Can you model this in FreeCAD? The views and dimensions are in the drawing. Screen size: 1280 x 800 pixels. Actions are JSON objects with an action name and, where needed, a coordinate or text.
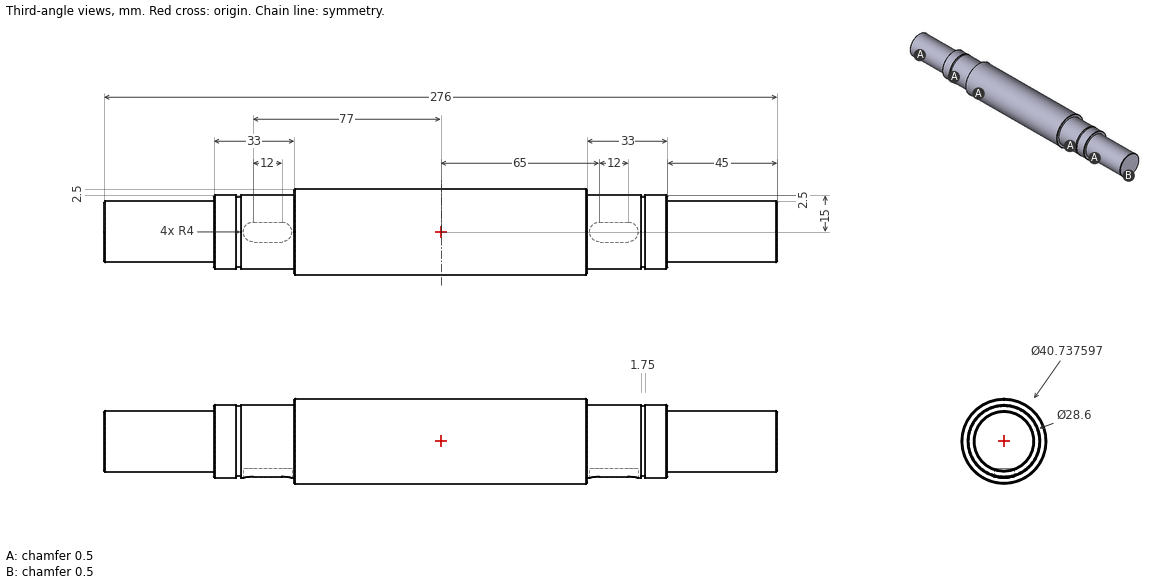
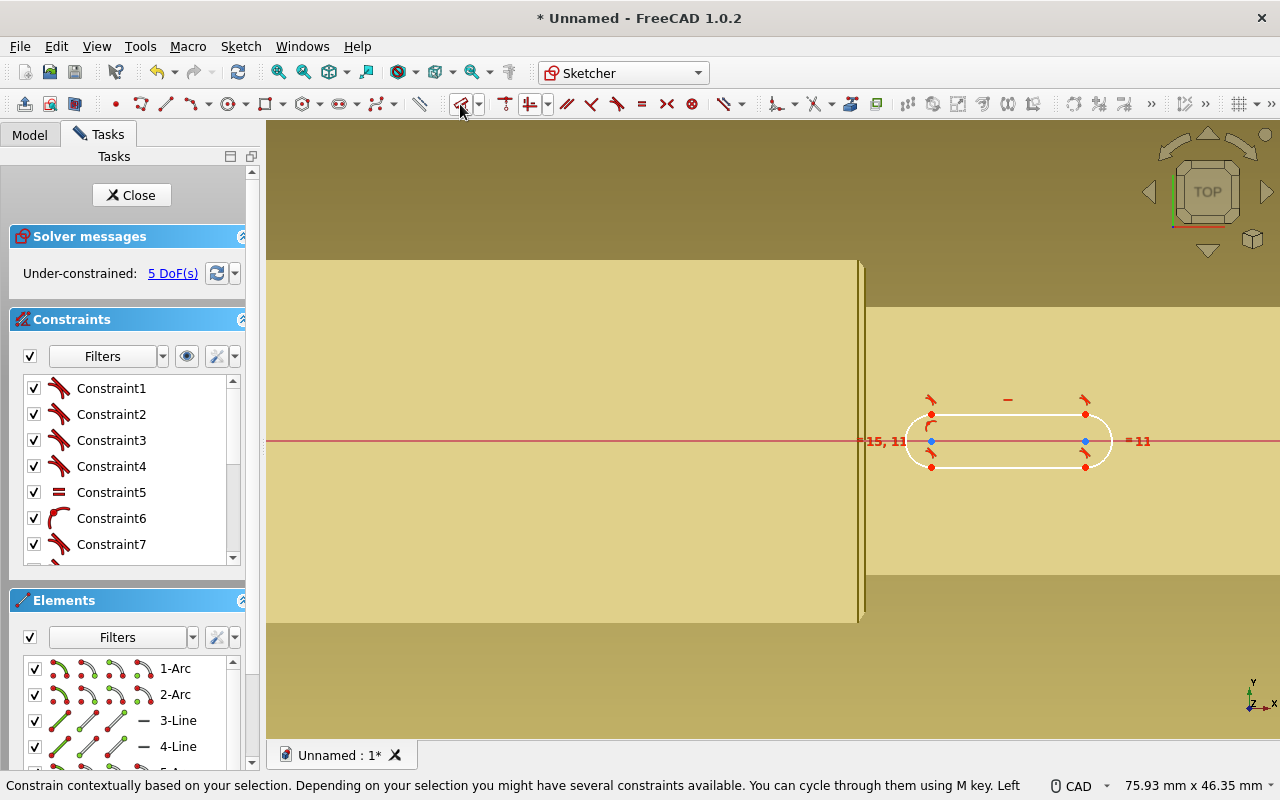
{"action": "scroll", "coordinate": [914, 426], "scroll_direction": "down", "scroll_amount": 7}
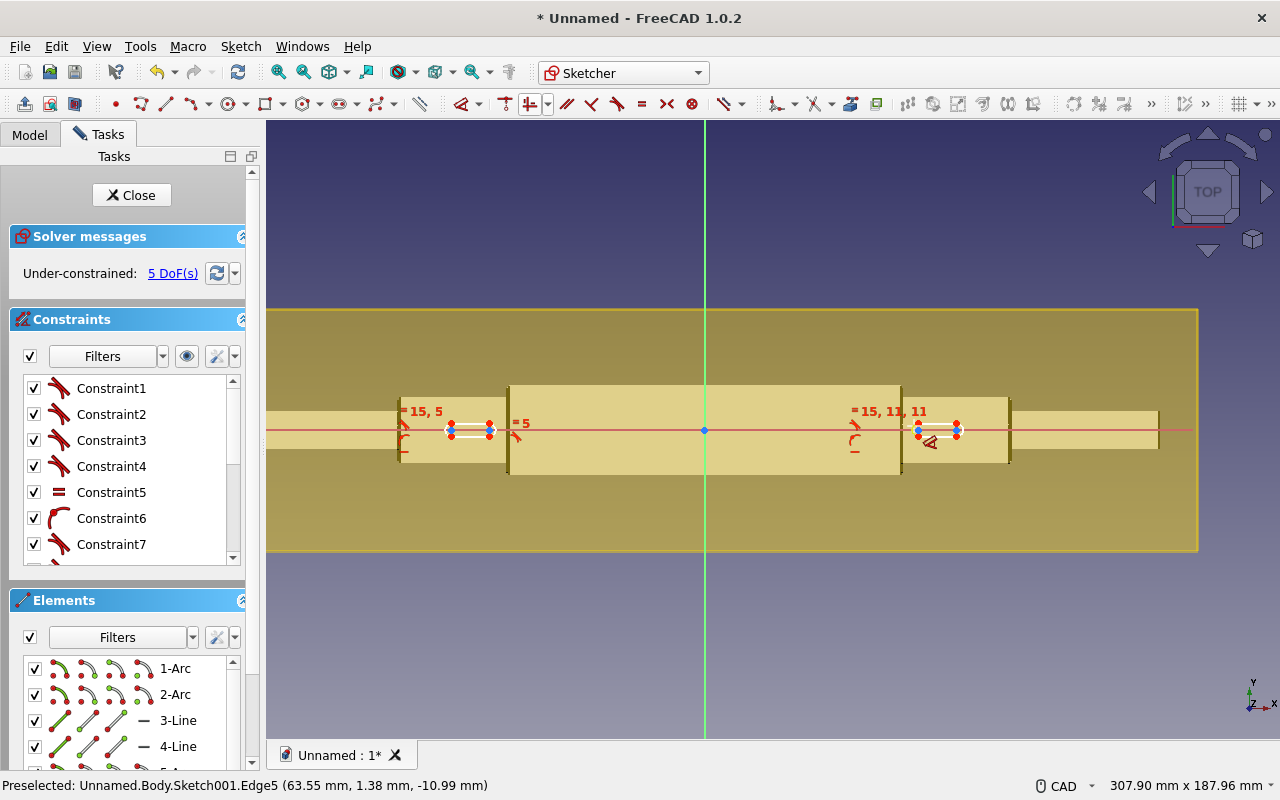
{"action": "scroll", "coordinate": [447, 426], "scroll_direction": "up", "scroll_amount": 7}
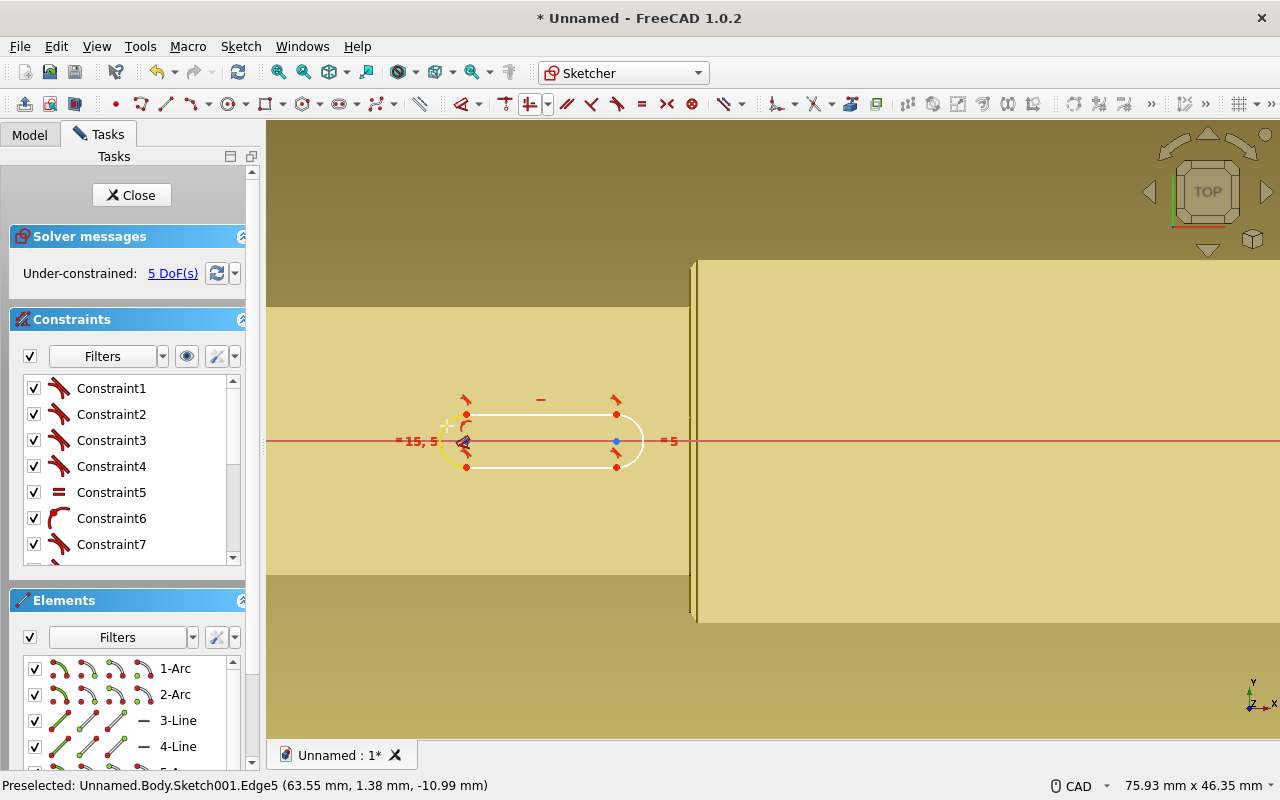
{"action": "left_click", "coordinate": [445, 426]}
{"action": "left_click", "coordinate": [419, 408]}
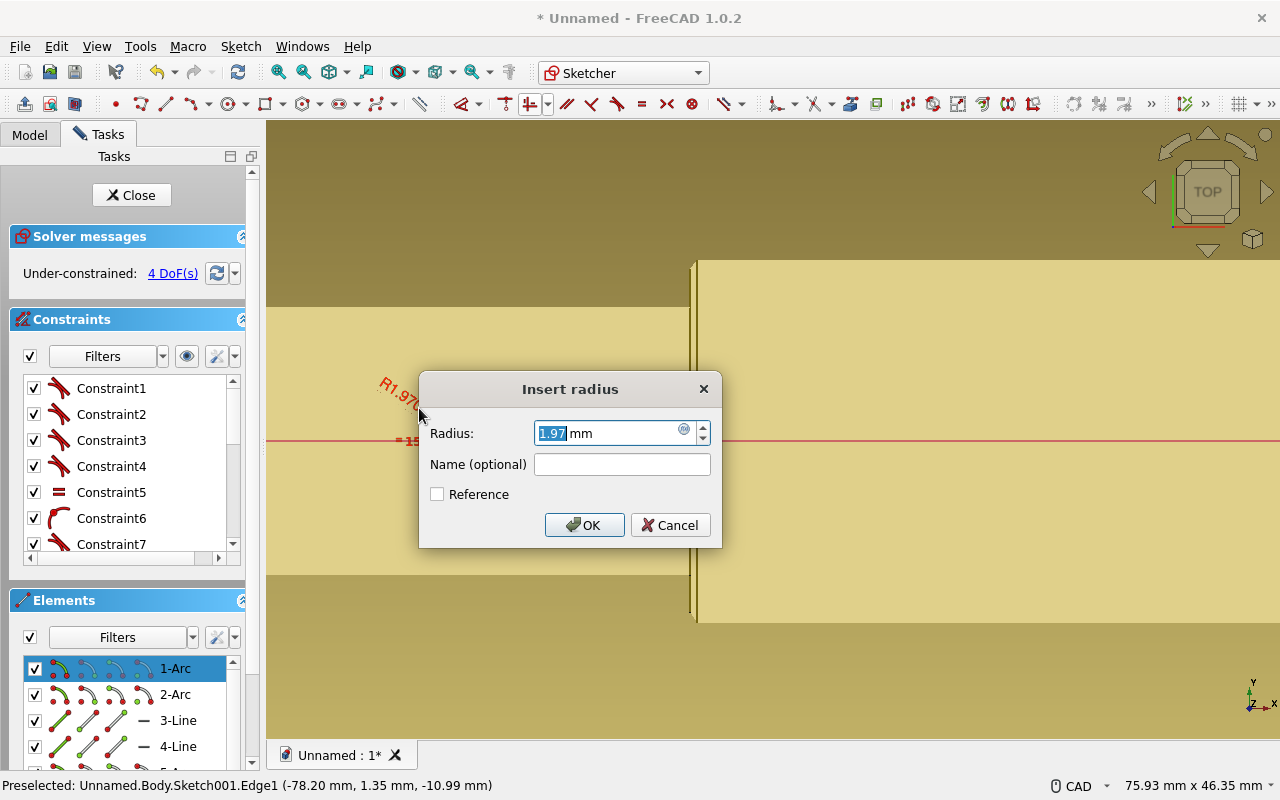
{"action": "type", "text": "4"}
{"action": "key", "text": "Return"}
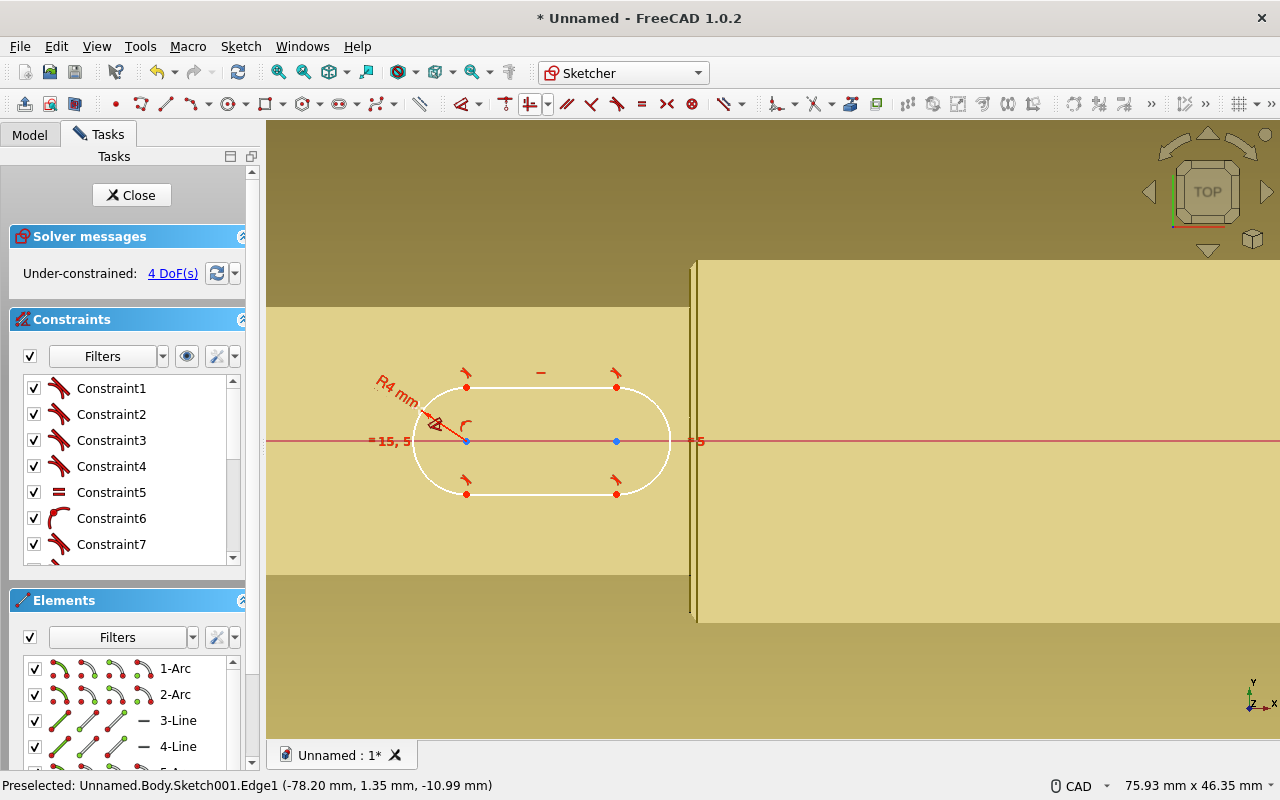
{"action": "scroll", "coordinate": [447, 426], "scroll_direction": "down", "scroll_amount": 7}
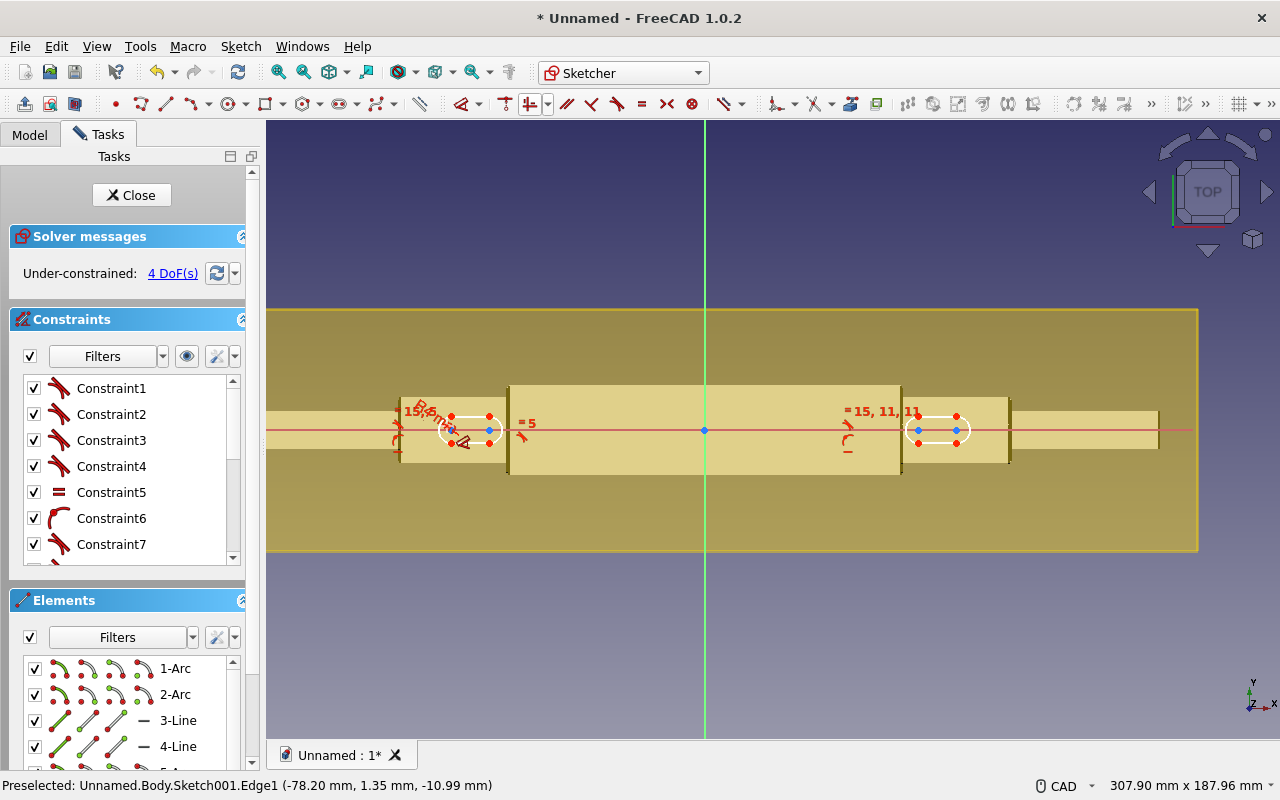
{"action": "scroll", "coordinate": [463, 417], "scroll_direction": "up", "scroll_amount": 2}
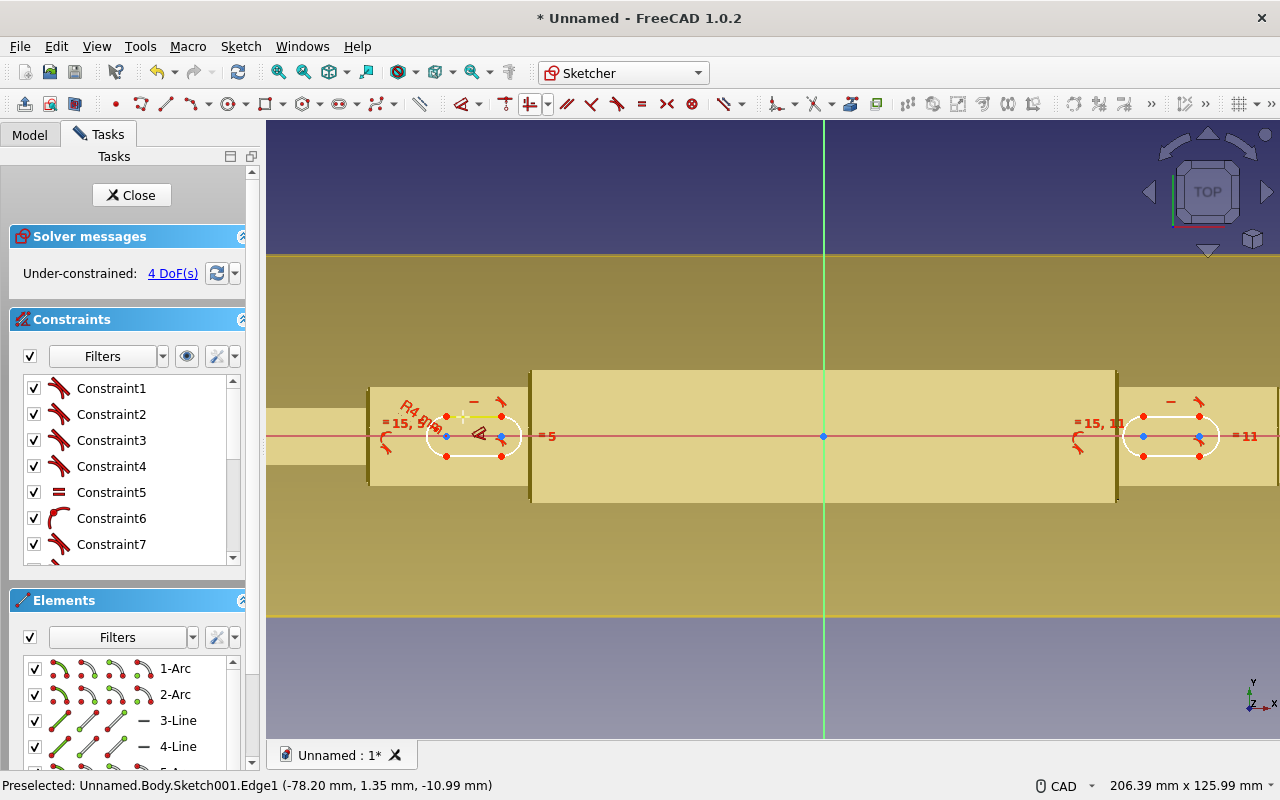
{"action": "left_click", "coordinate": [463, 417]}
{"action": "left_click", "coordinate": [474, 383]}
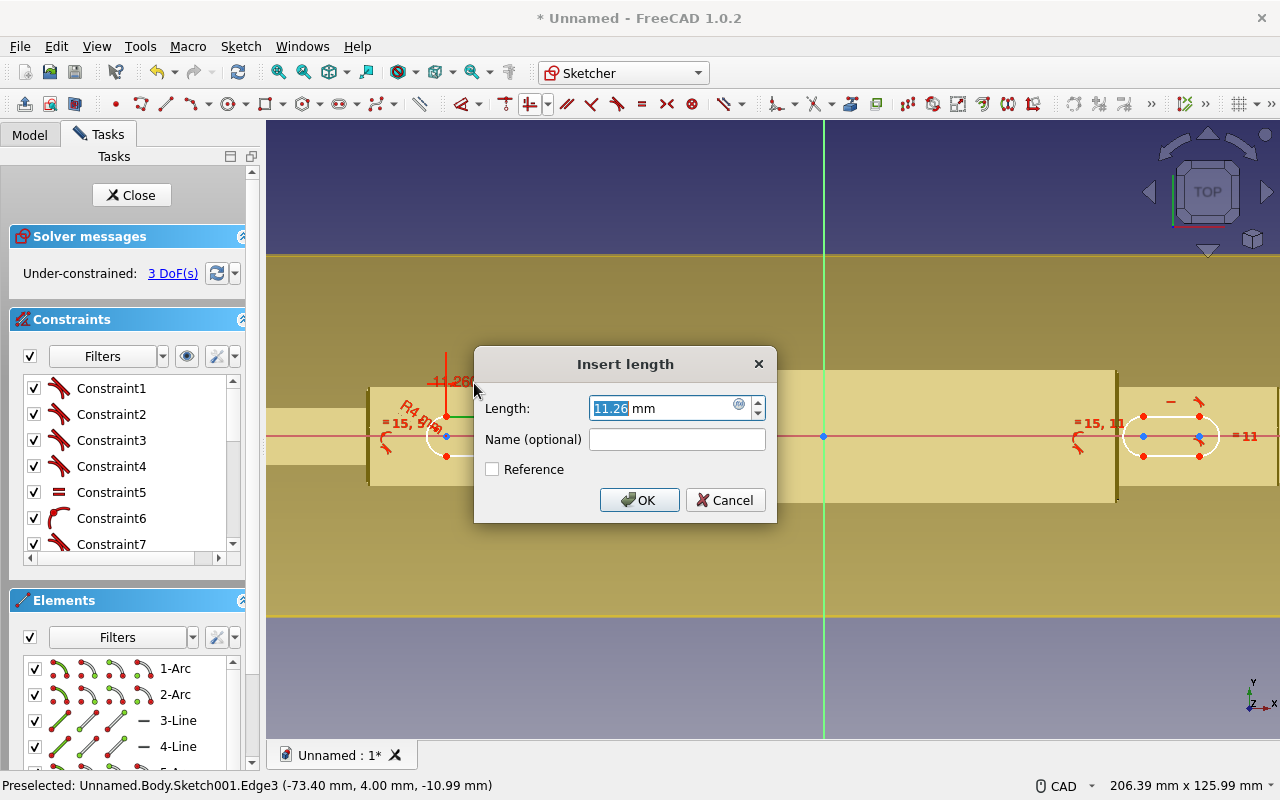
{"action": "type", "text": "12"}
{"action": "key", "text": "Return"}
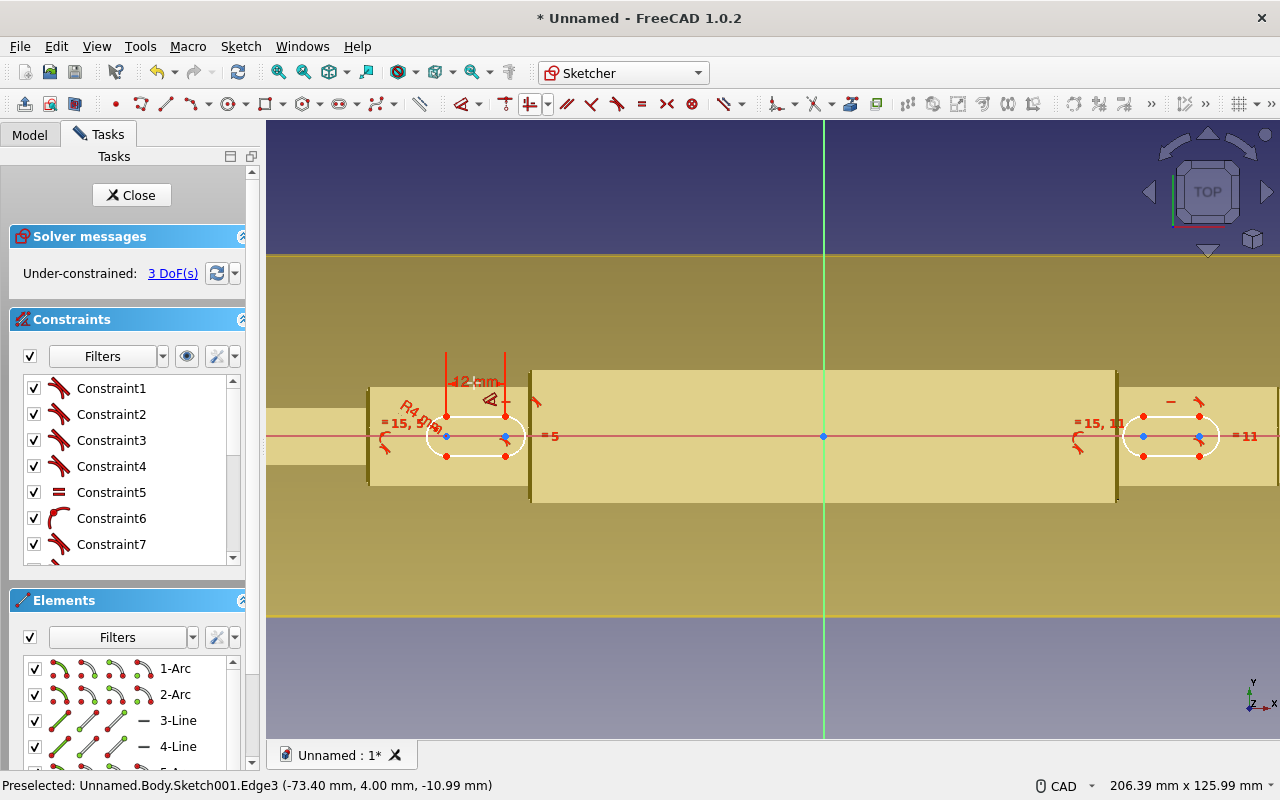
{"action": "scroll", "coordinate": [462, 416], "scroll_direction": "down", "scroll_amount": 2}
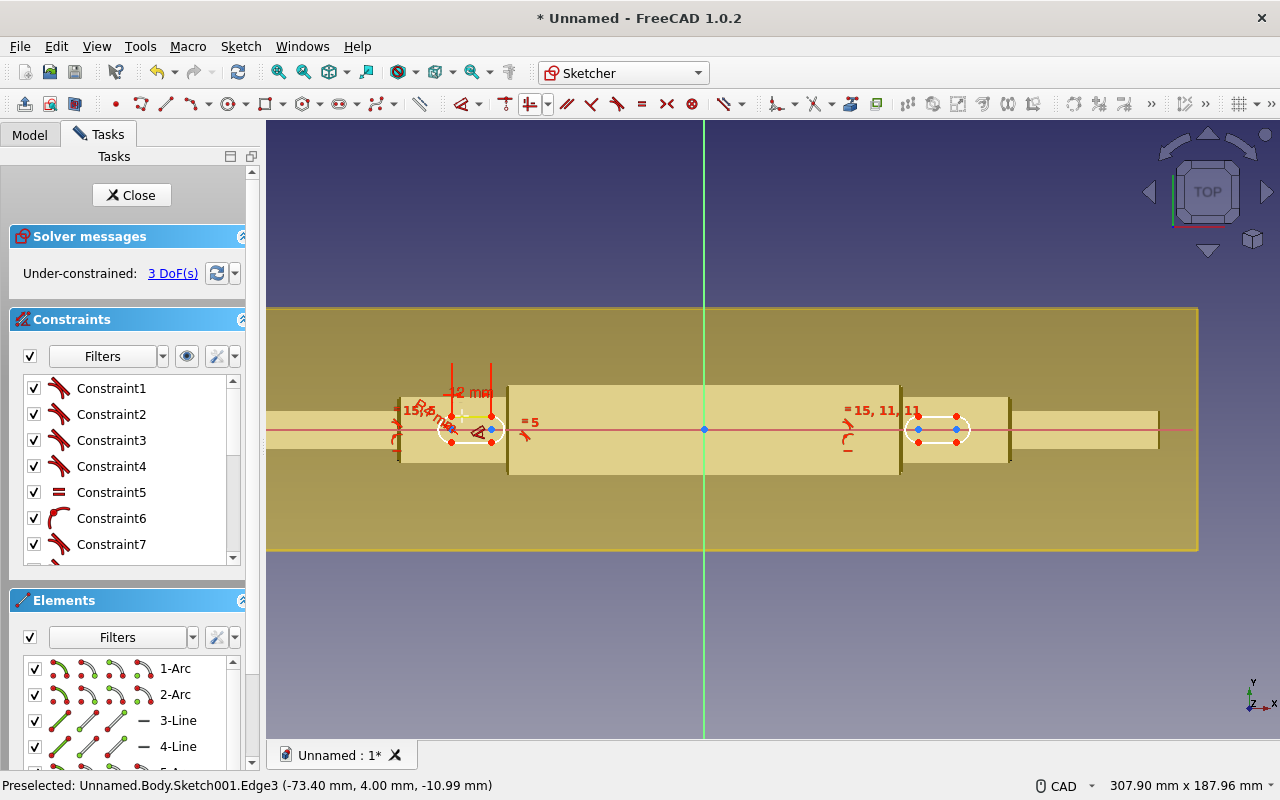
{"action": "left_click", "coordinate": [930, 417]}
{"action": "left_click", "coordinate": [938, 383]}